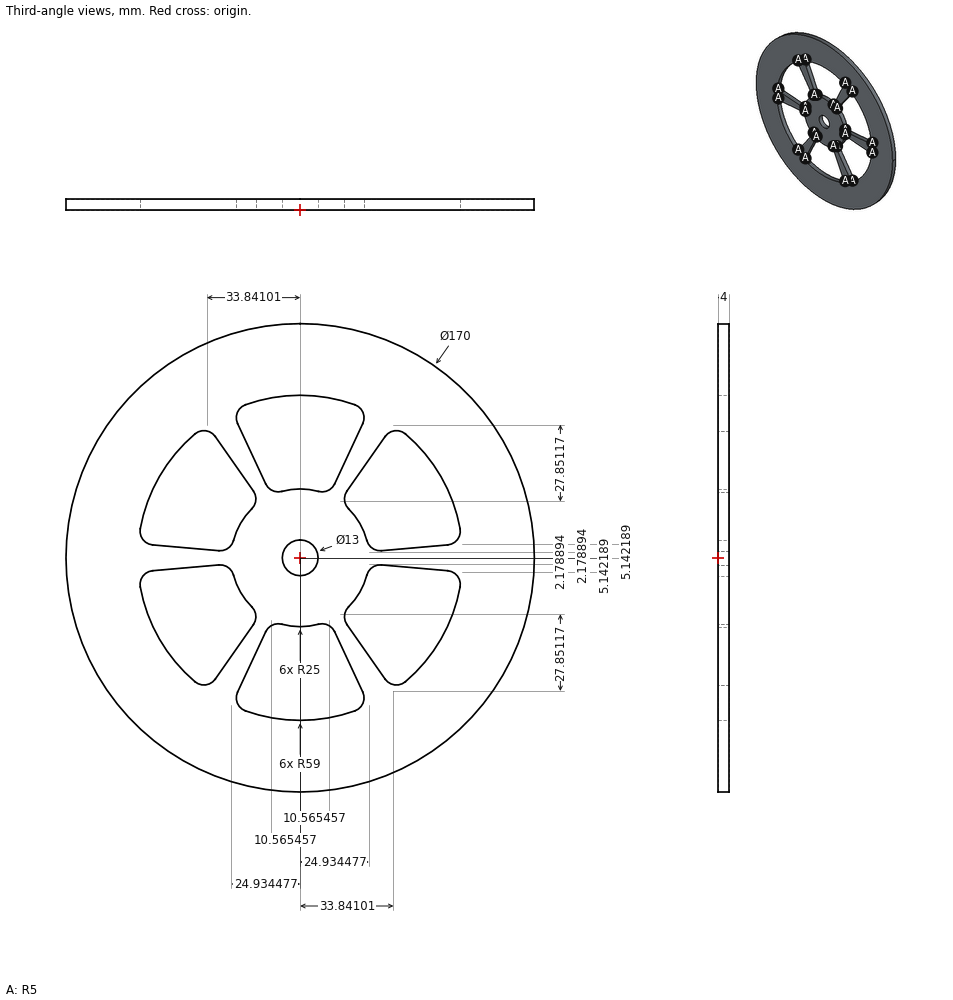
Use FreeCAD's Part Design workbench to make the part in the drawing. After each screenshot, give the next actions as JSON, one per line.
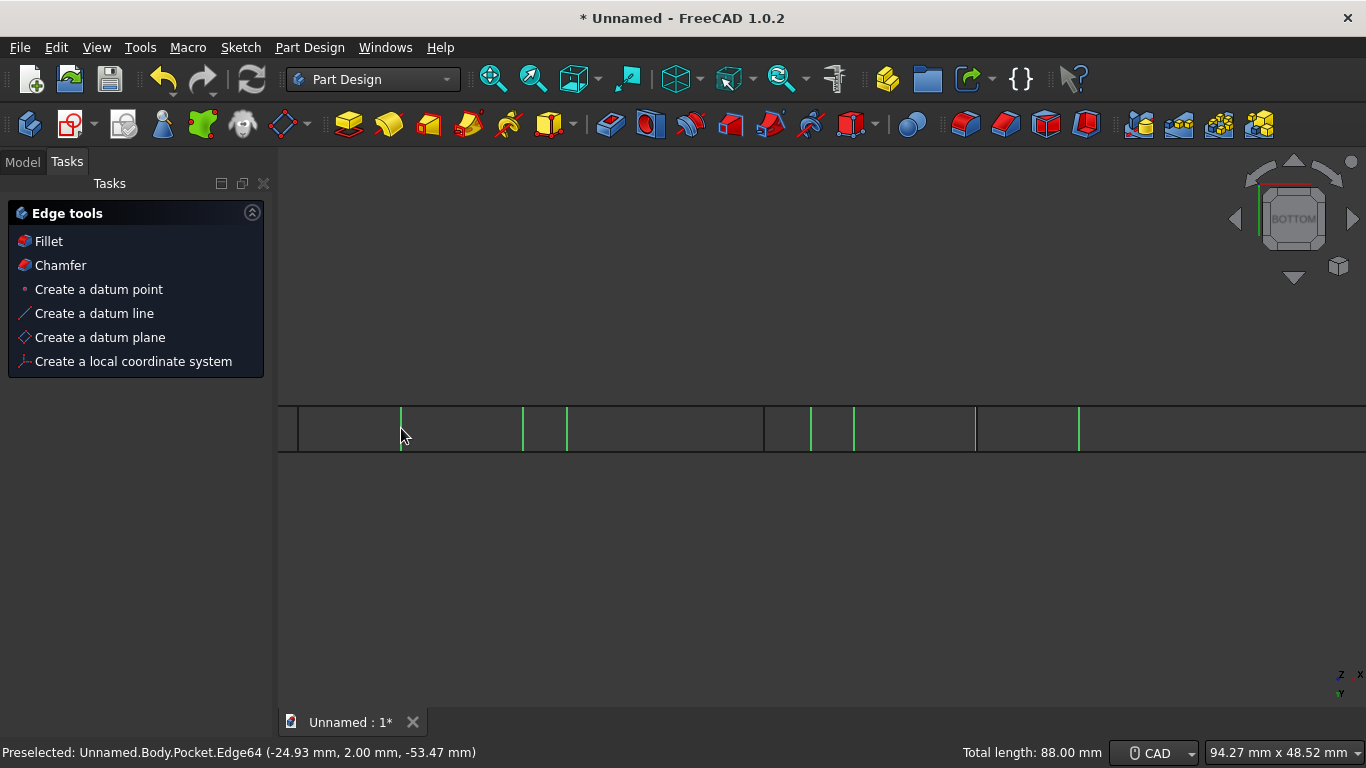
{"action": "left_click", "coordinate": [977, 428], "text": "ctrl"}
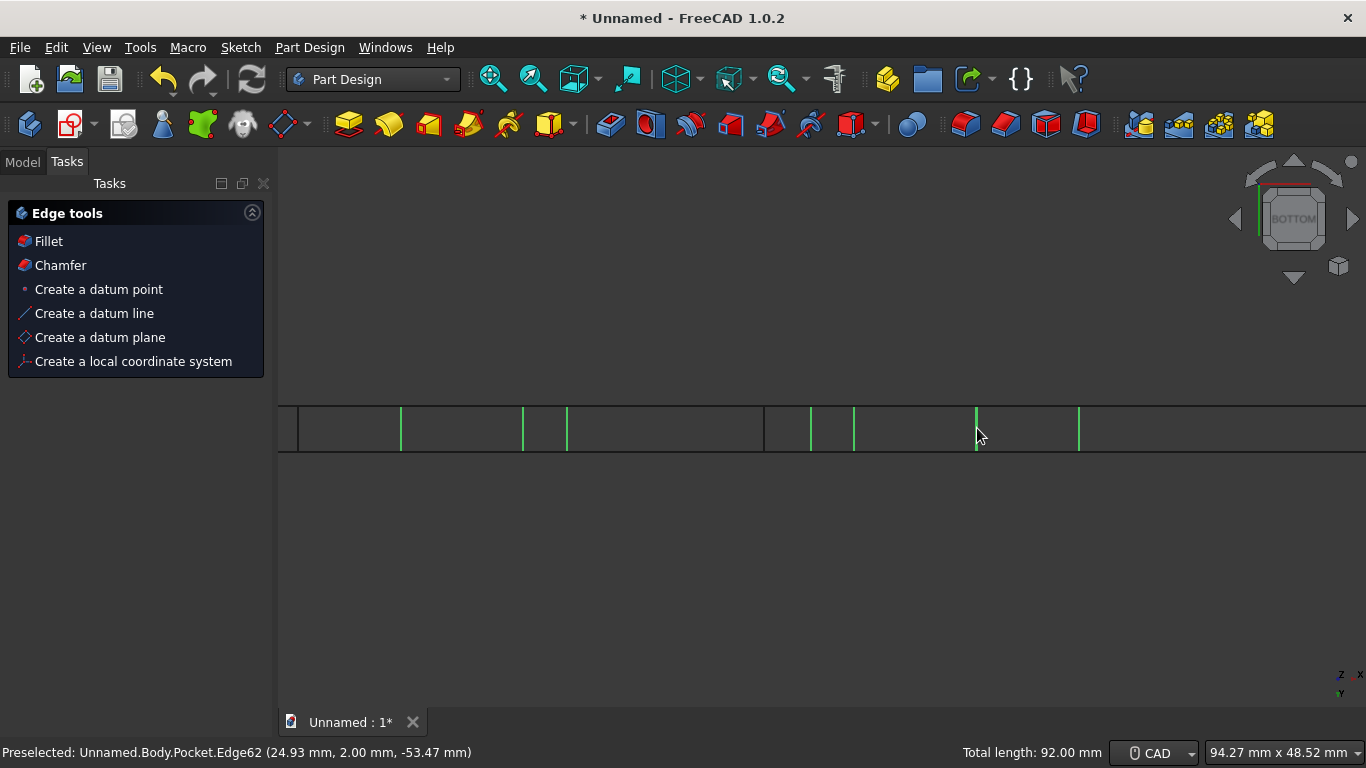
{"action": "left_click", "coordinate": [494, 80]}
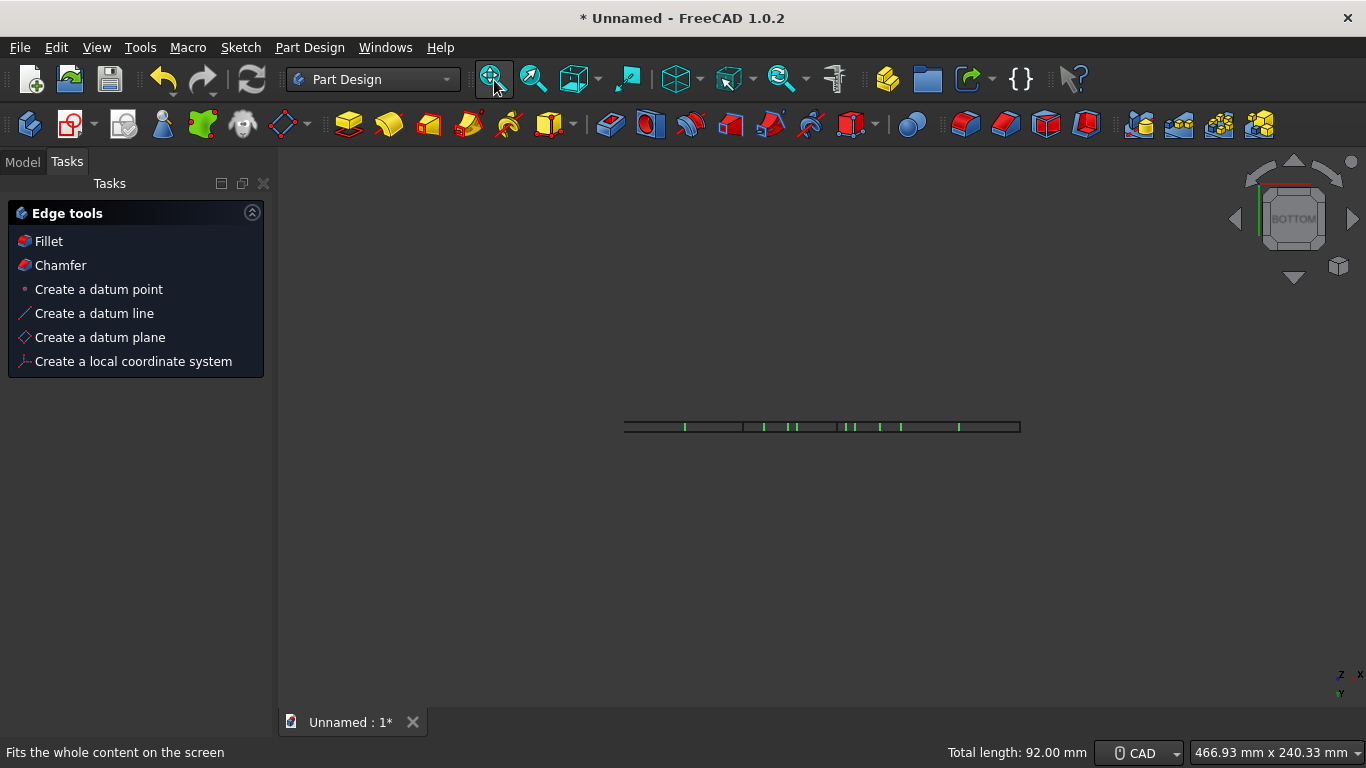
{"action": "key", "text": "4"}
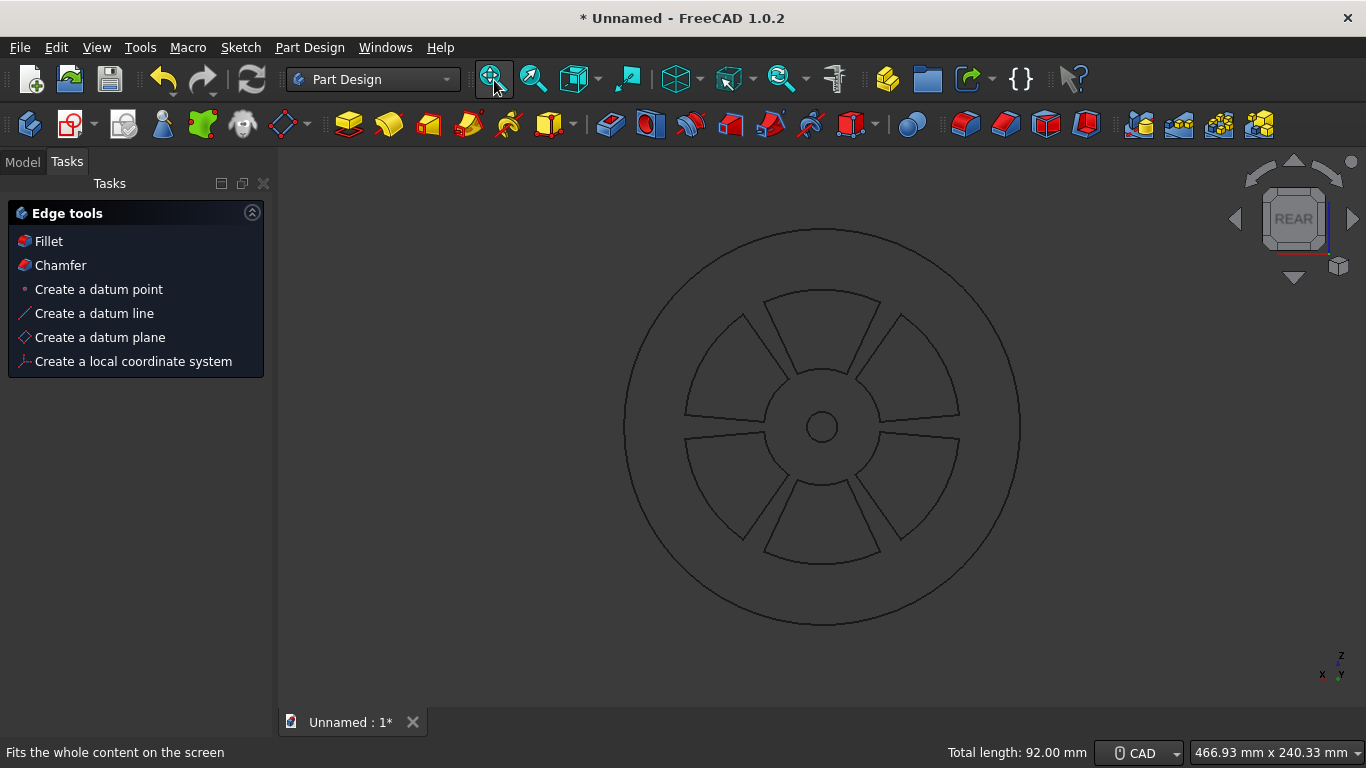
{"action": "scroll", "coordinate": [901, 539], "scroll_direction": "up", "scroll_amount": 8}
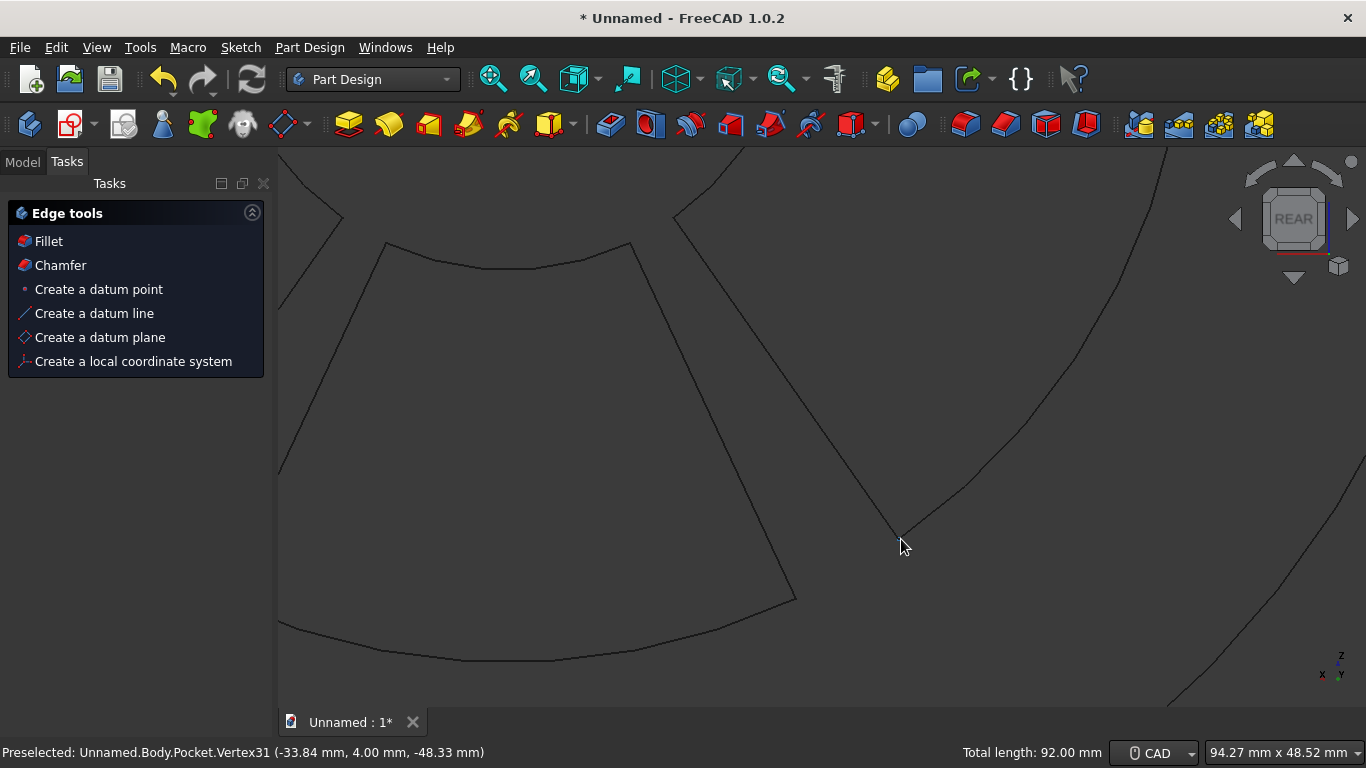
{"action": "left_click", "coordinate": [494, 80]}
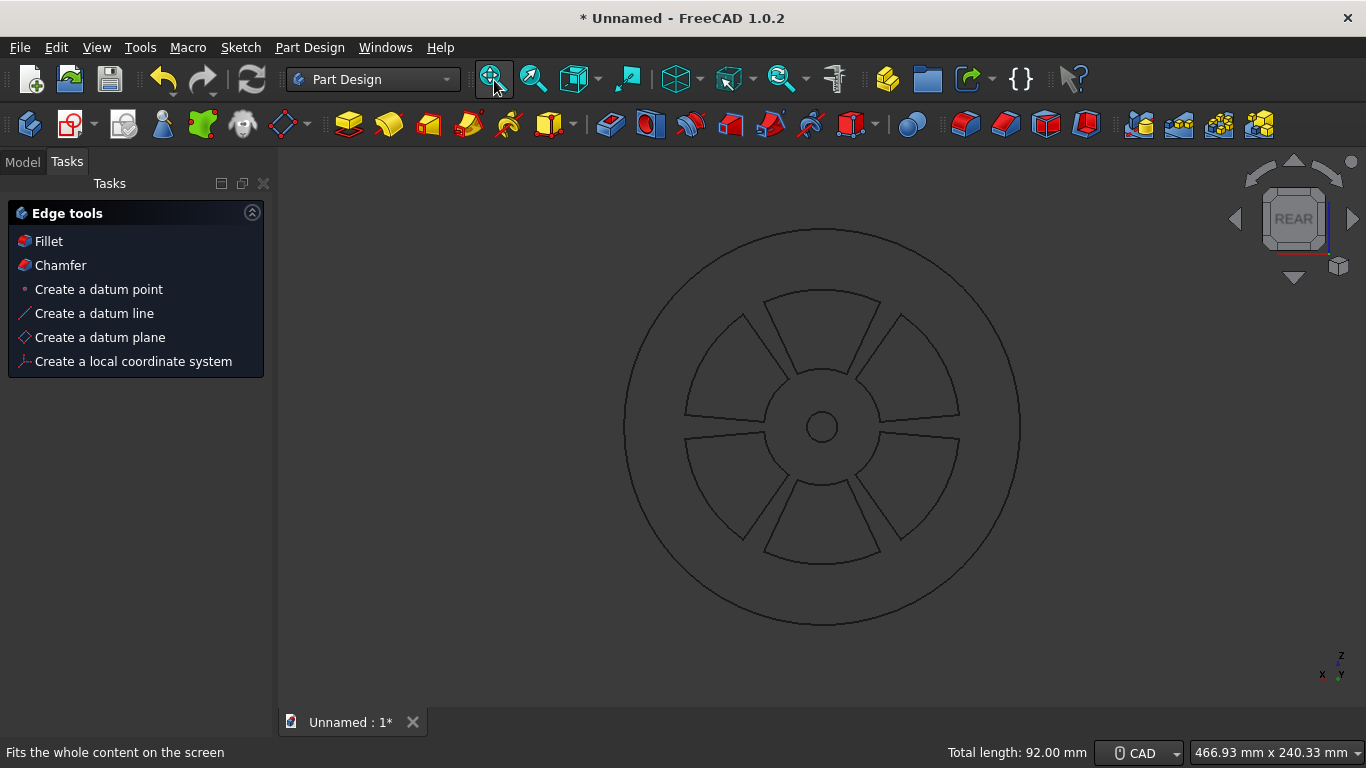
{"action": "key", "text": "6"}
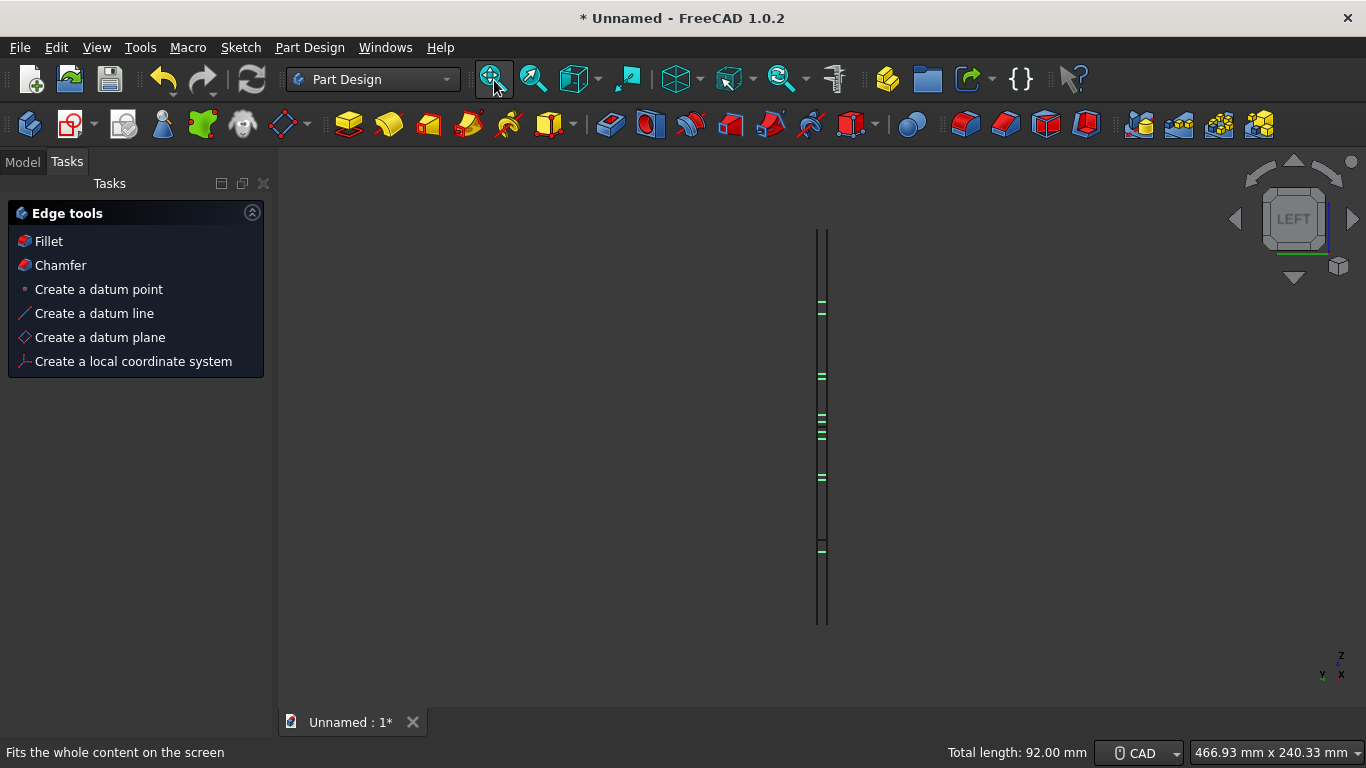
{"action": "scroll", "coordinate": [822, 539], "scroll_direction": "up", "scroll_amount": 8}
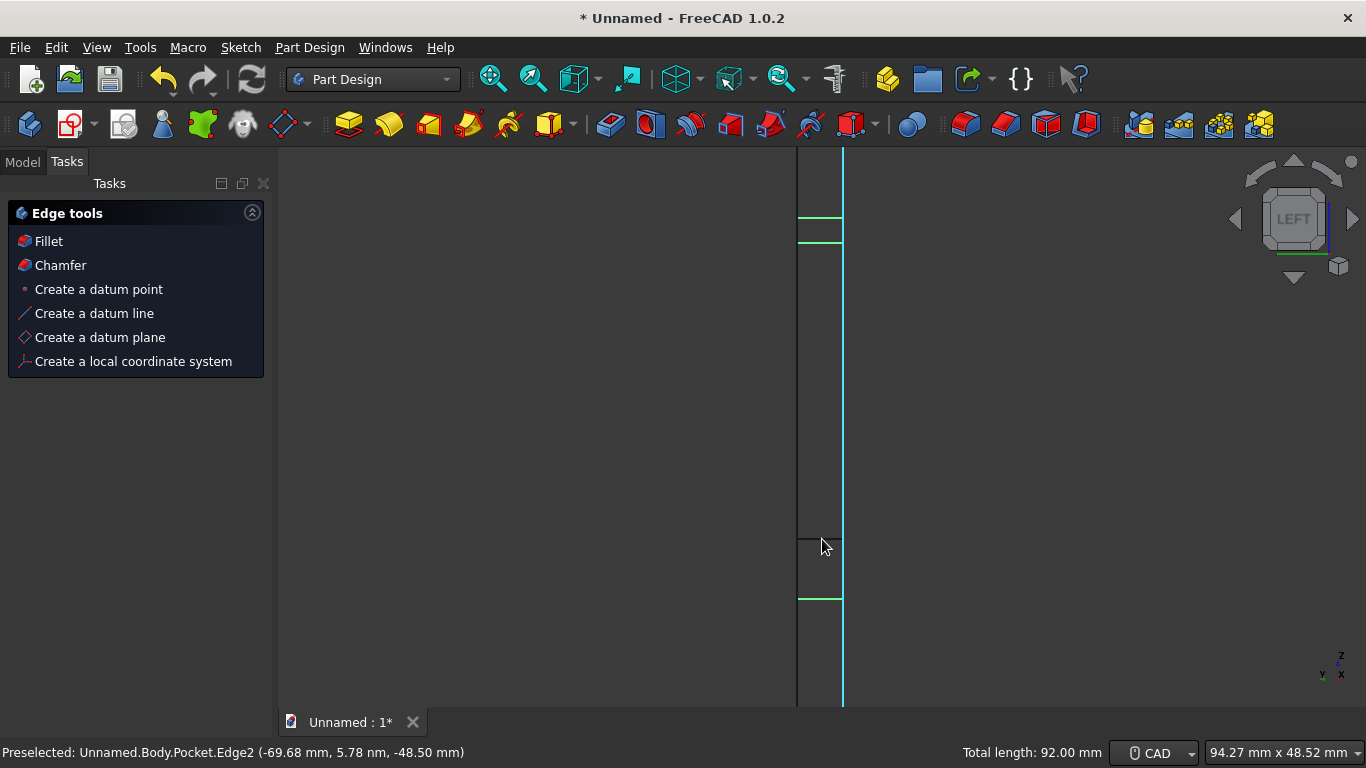
{"action": "left_click", "coordinate": [820, 538], "text": "ctrl"}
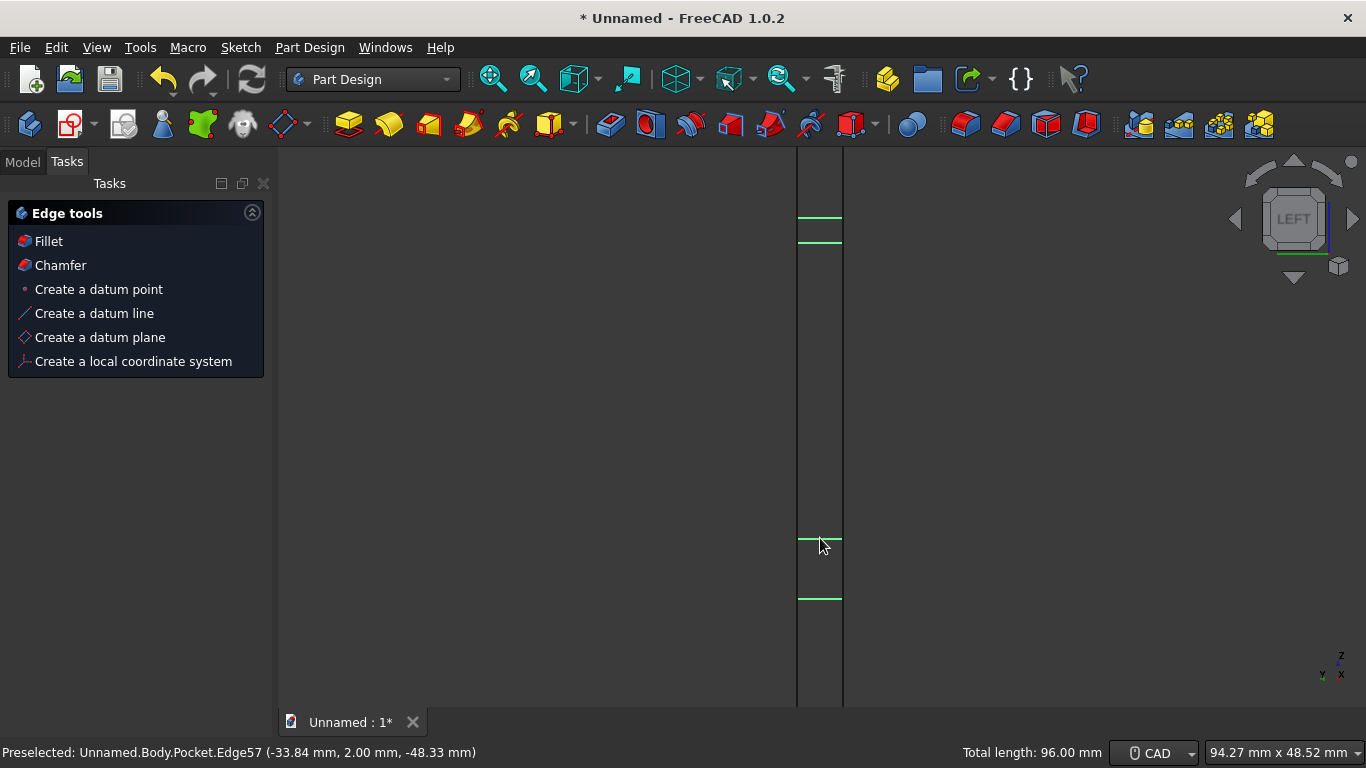
{"action": "key", "text": "v 1"}